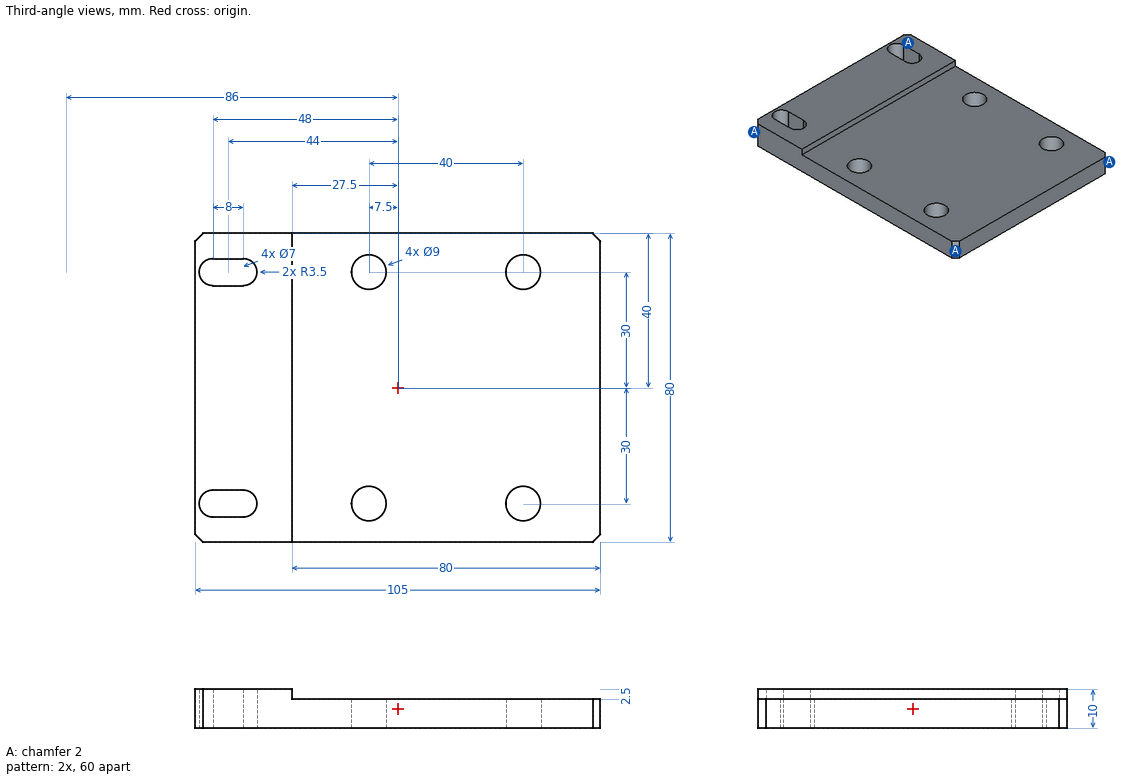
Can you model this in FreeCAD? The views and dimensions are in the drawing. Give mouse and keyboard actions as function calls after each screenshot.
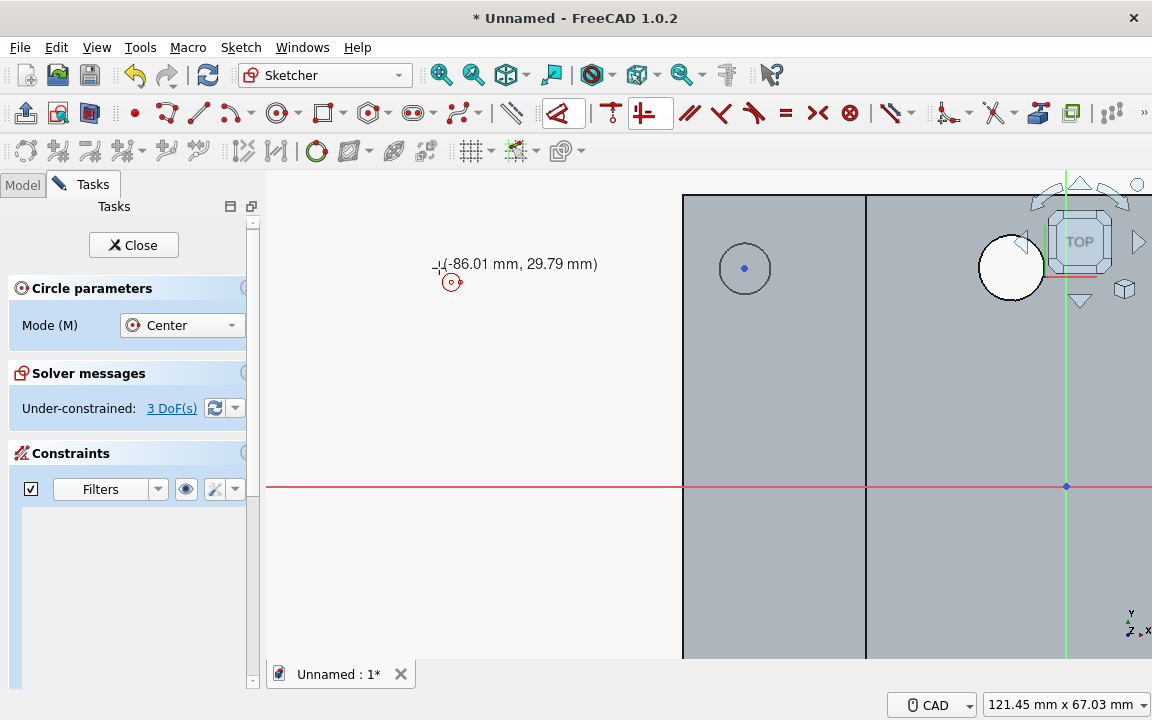
click(439, 268)
click(457, 250)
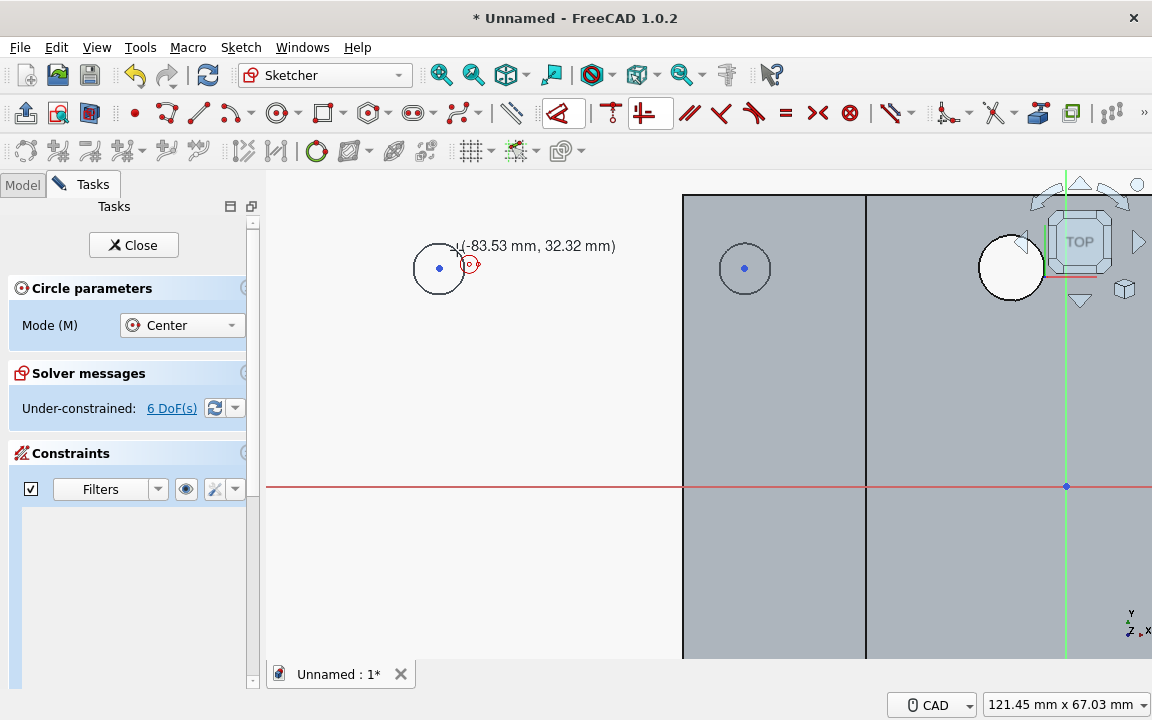
scroll(438, 268, down, 2)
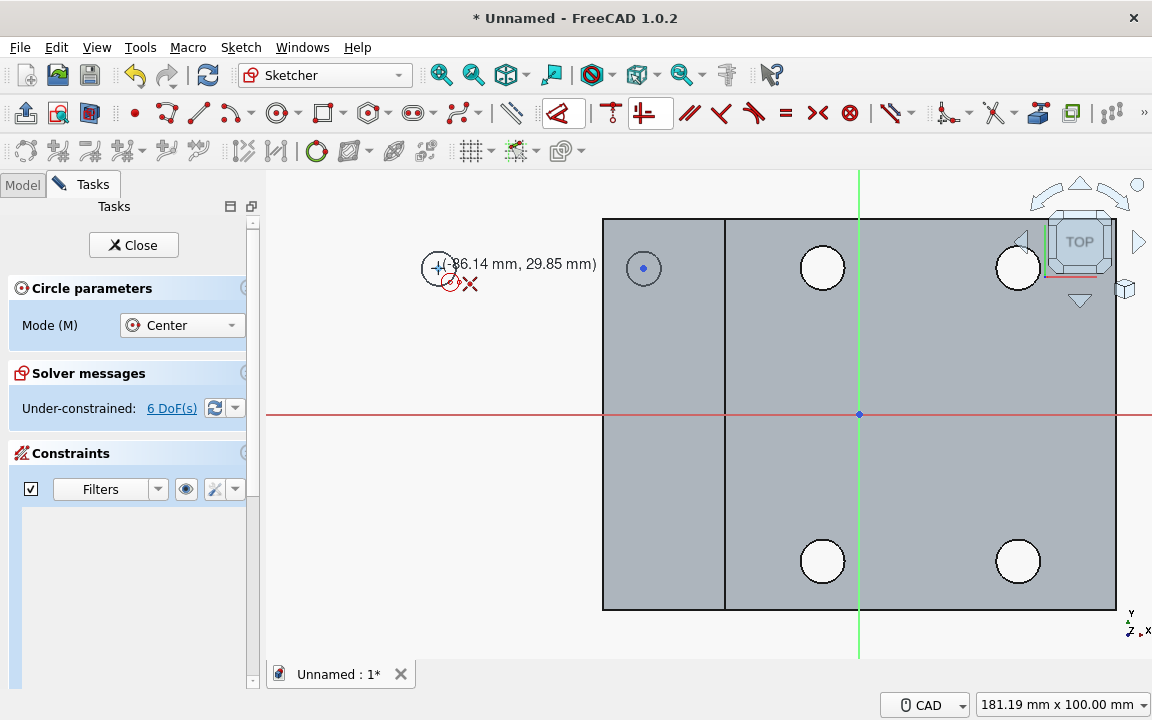
scroll(644, 561, up, 2)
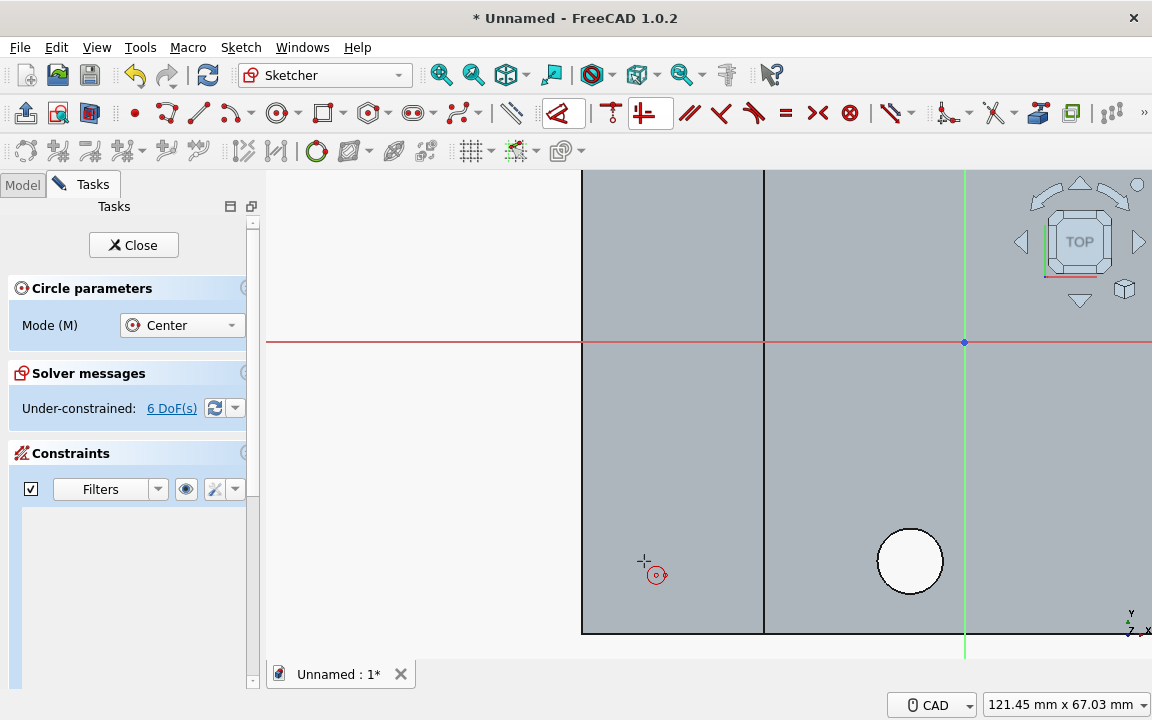
click(644, 561)
click(662, 543)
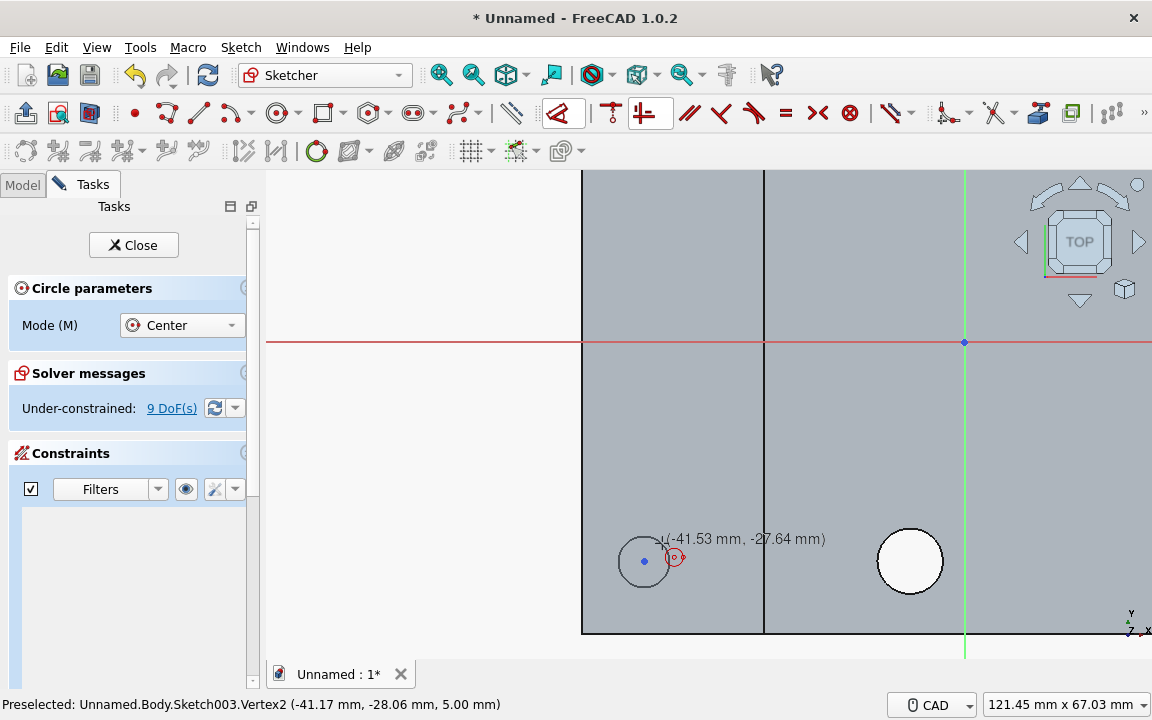
click(338, 561)
click(356, 543)
key(Escape)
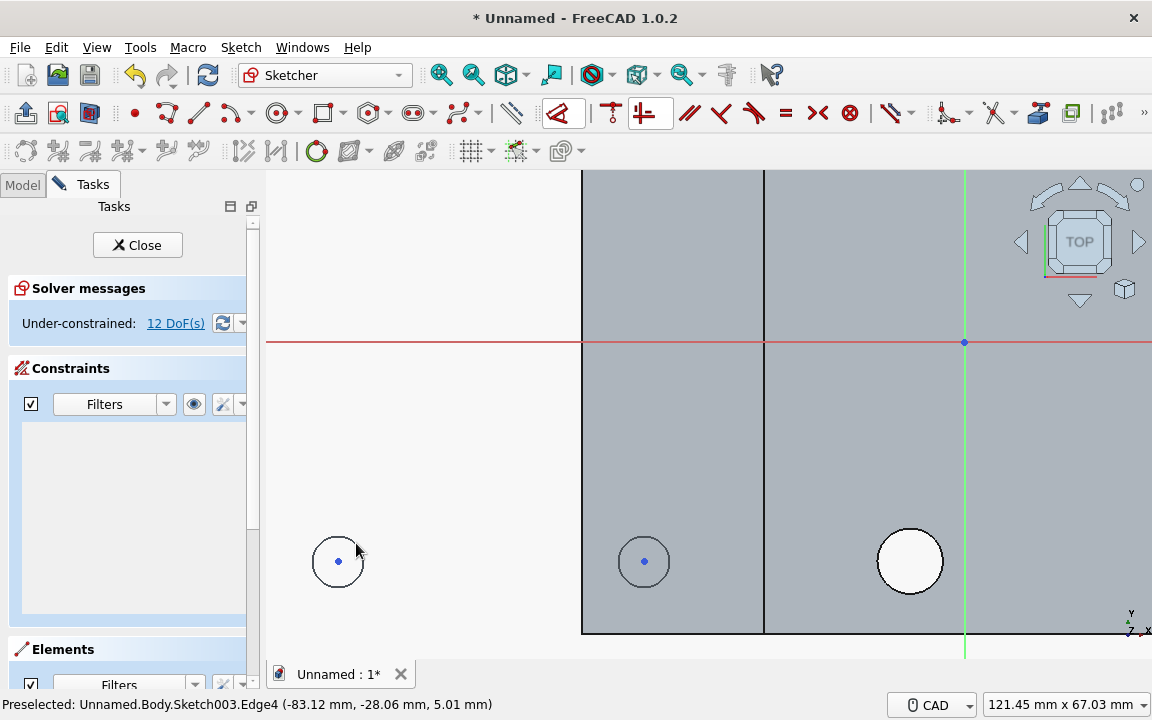
scroll(645, 561, down, 2)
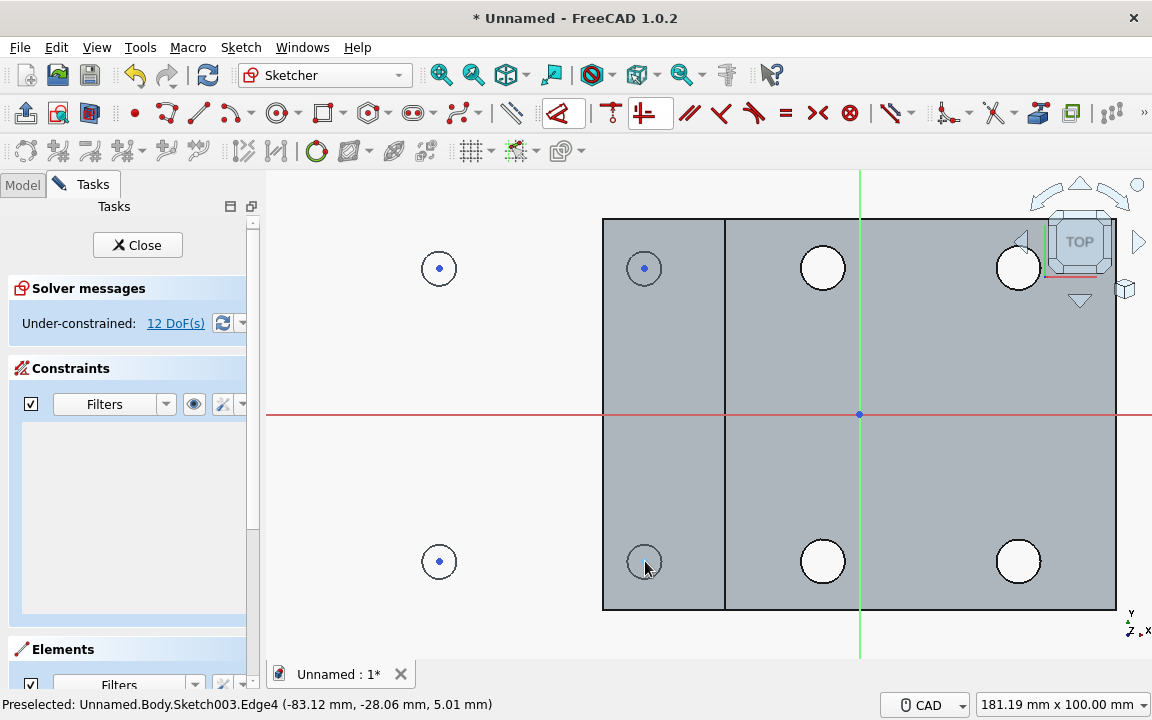
click(656, 257)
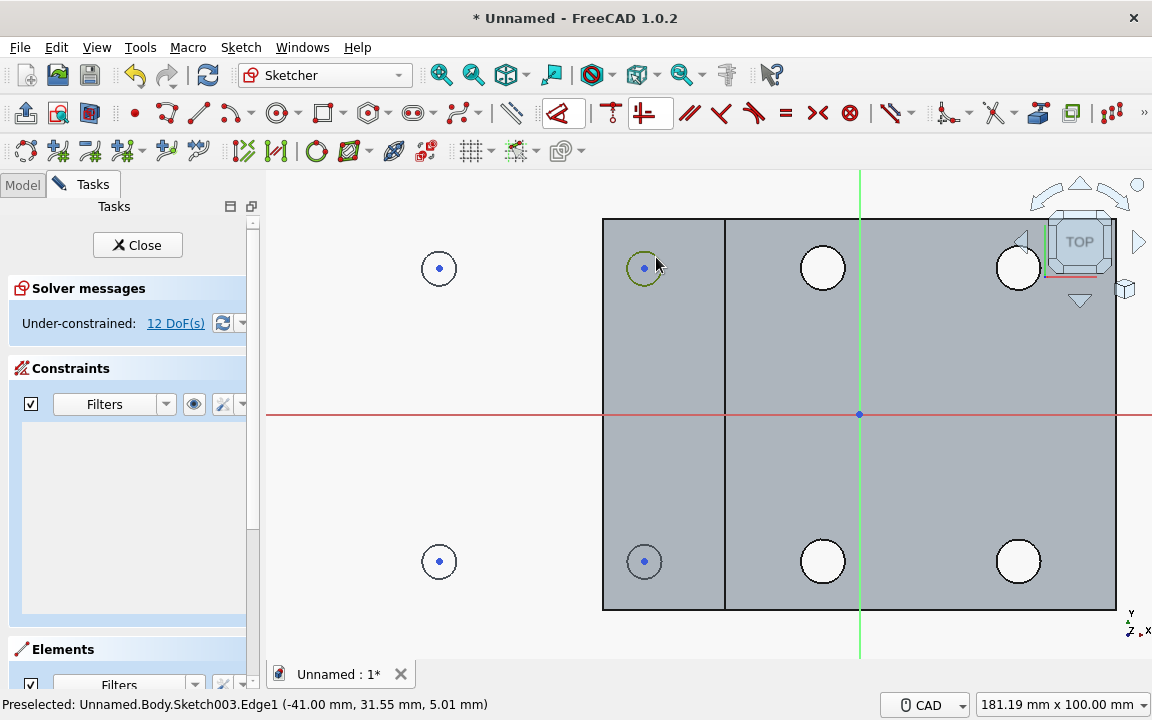
click(451, 257)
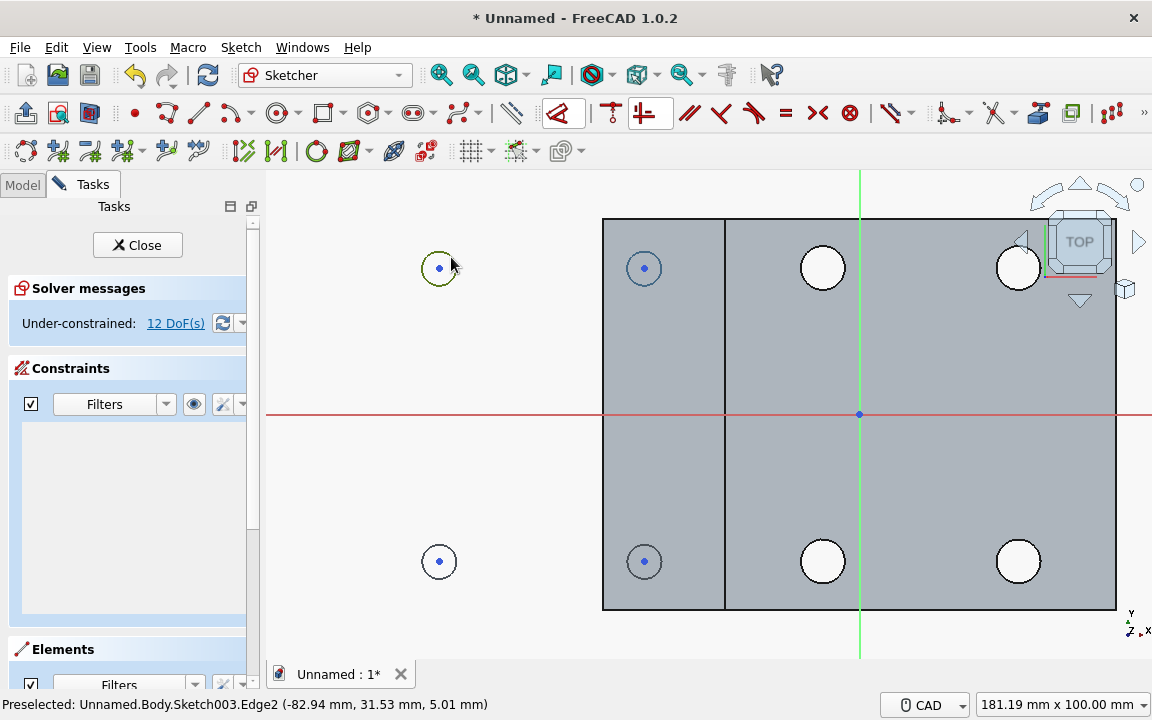
click(656, 550)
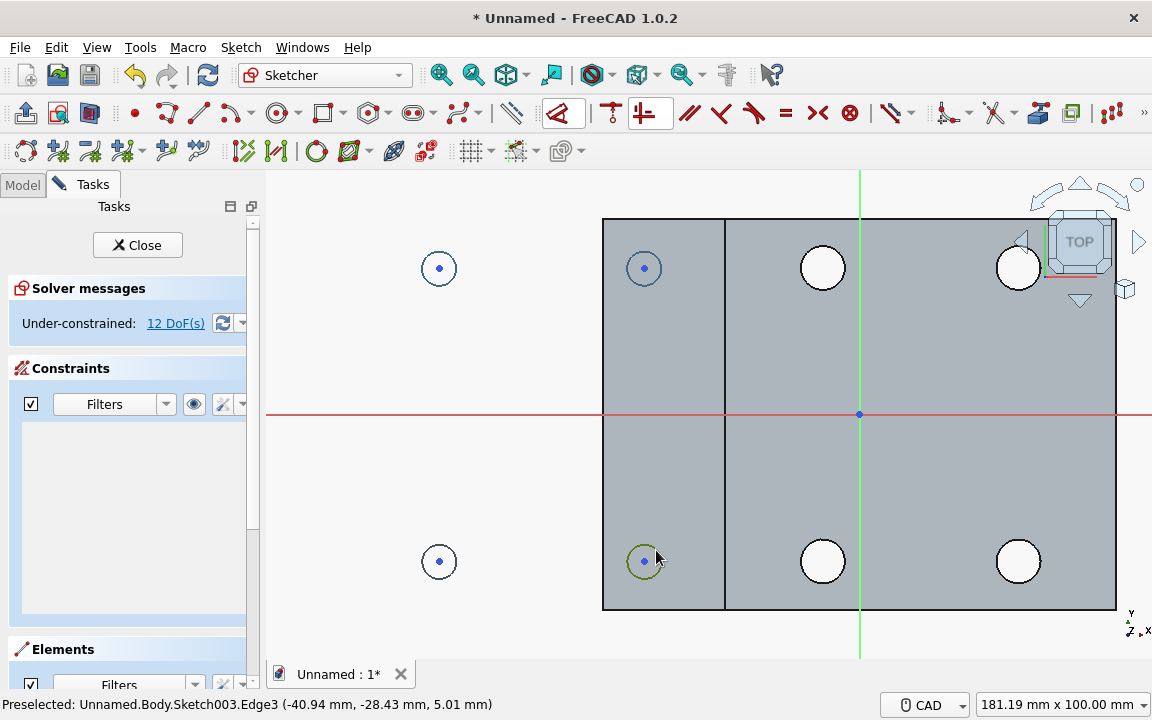
click(451, 550)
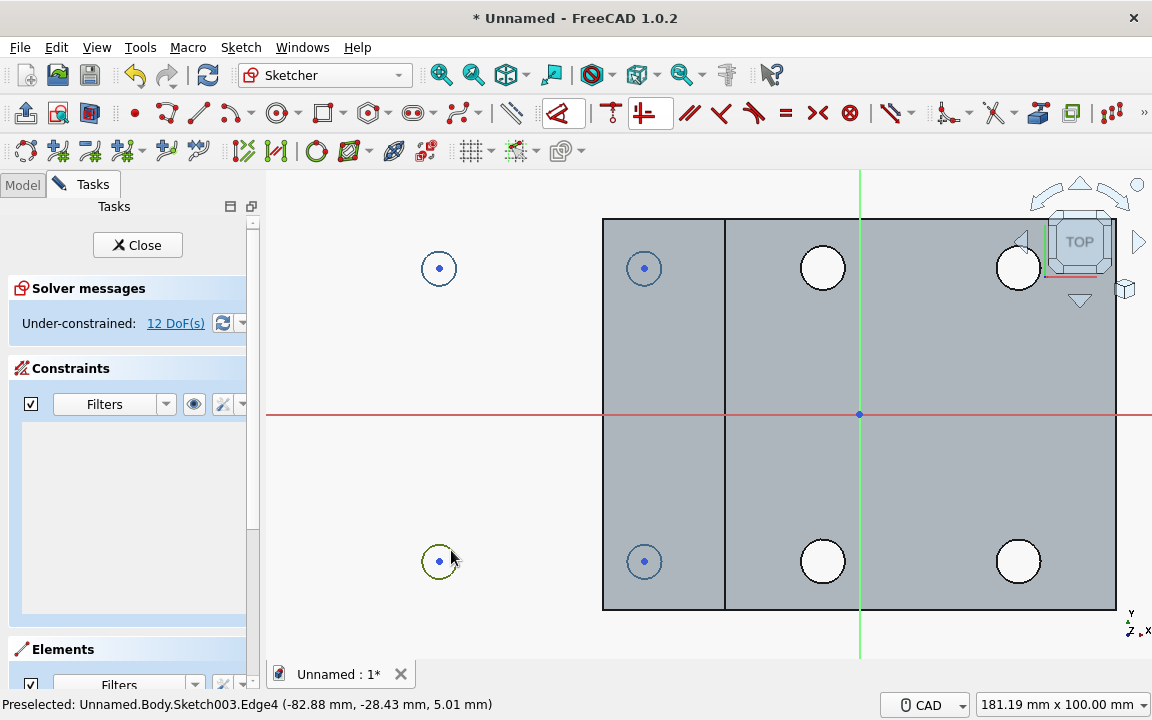
click(786, 114)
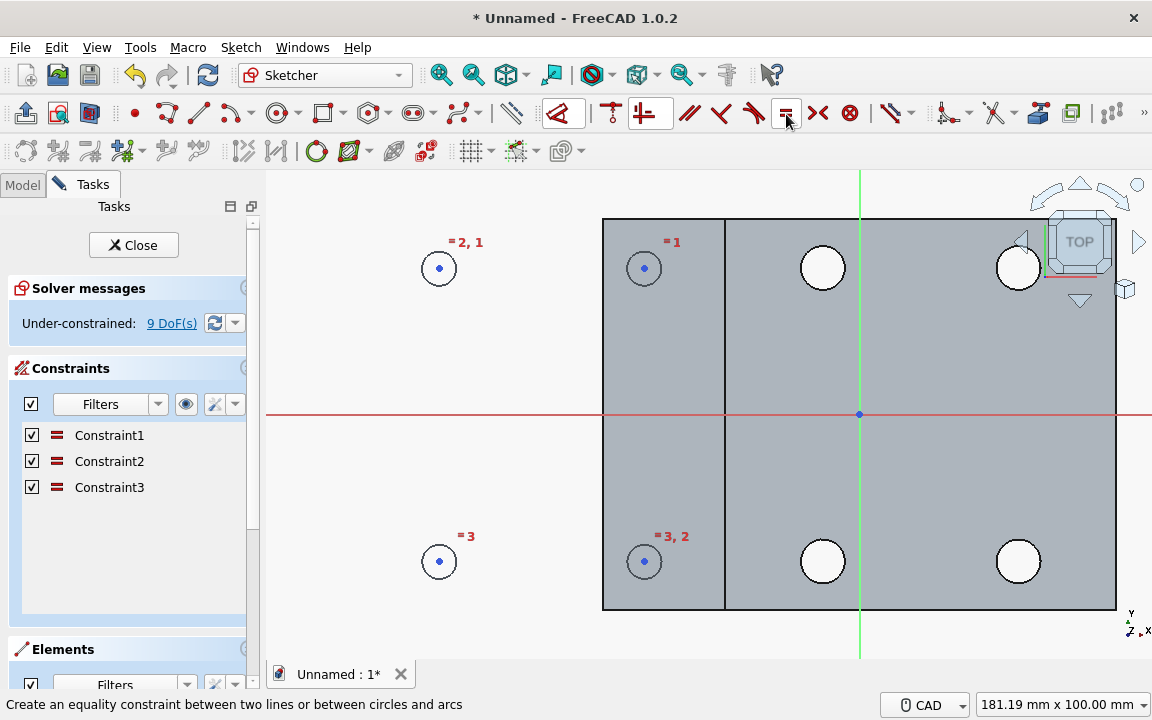
click(644, 269)